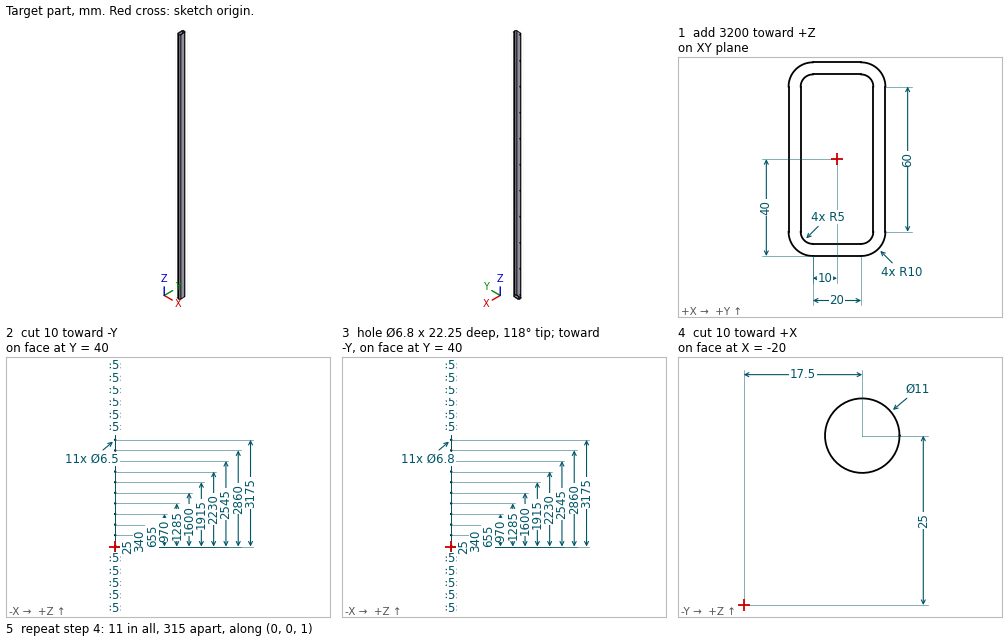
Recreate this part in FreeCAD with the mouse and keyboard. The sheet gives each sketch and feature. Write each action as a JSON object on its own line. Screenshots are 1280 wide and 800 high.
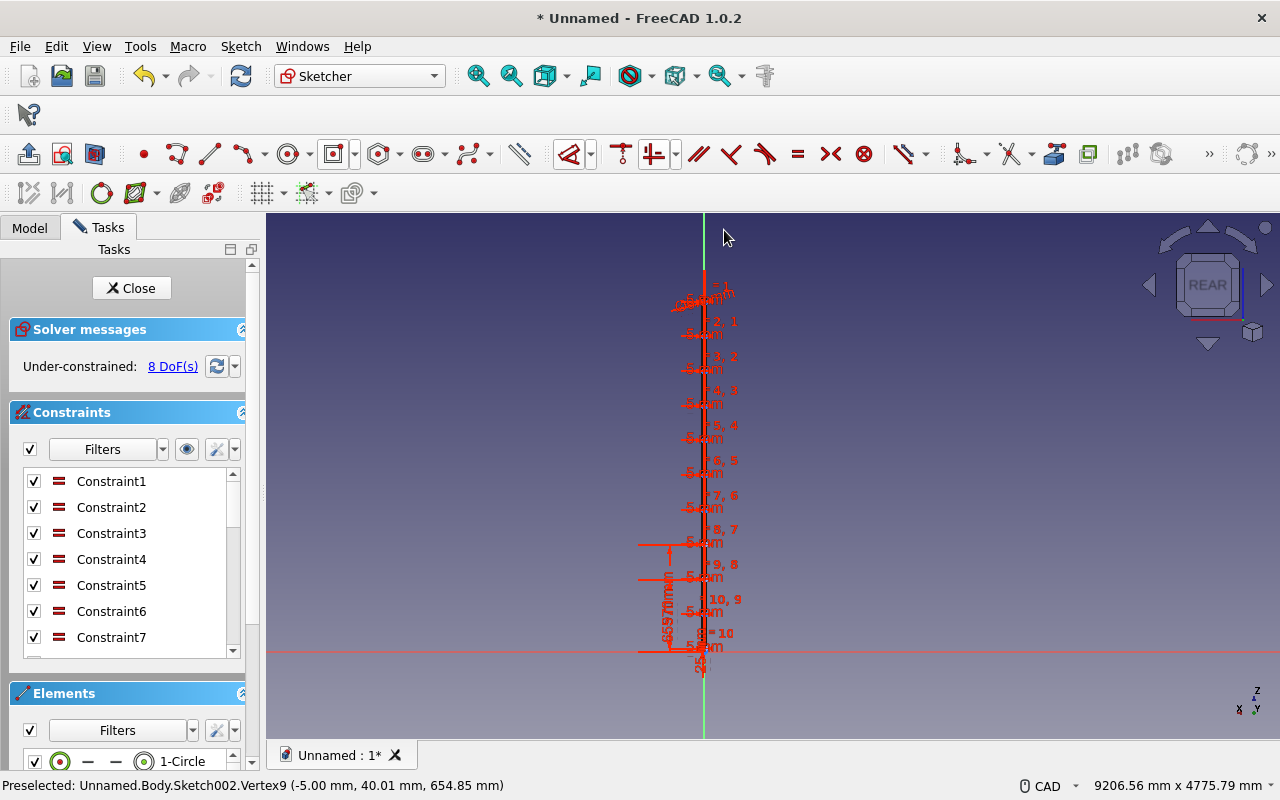
{"action": "left_click", "coordinate": [705, 614]}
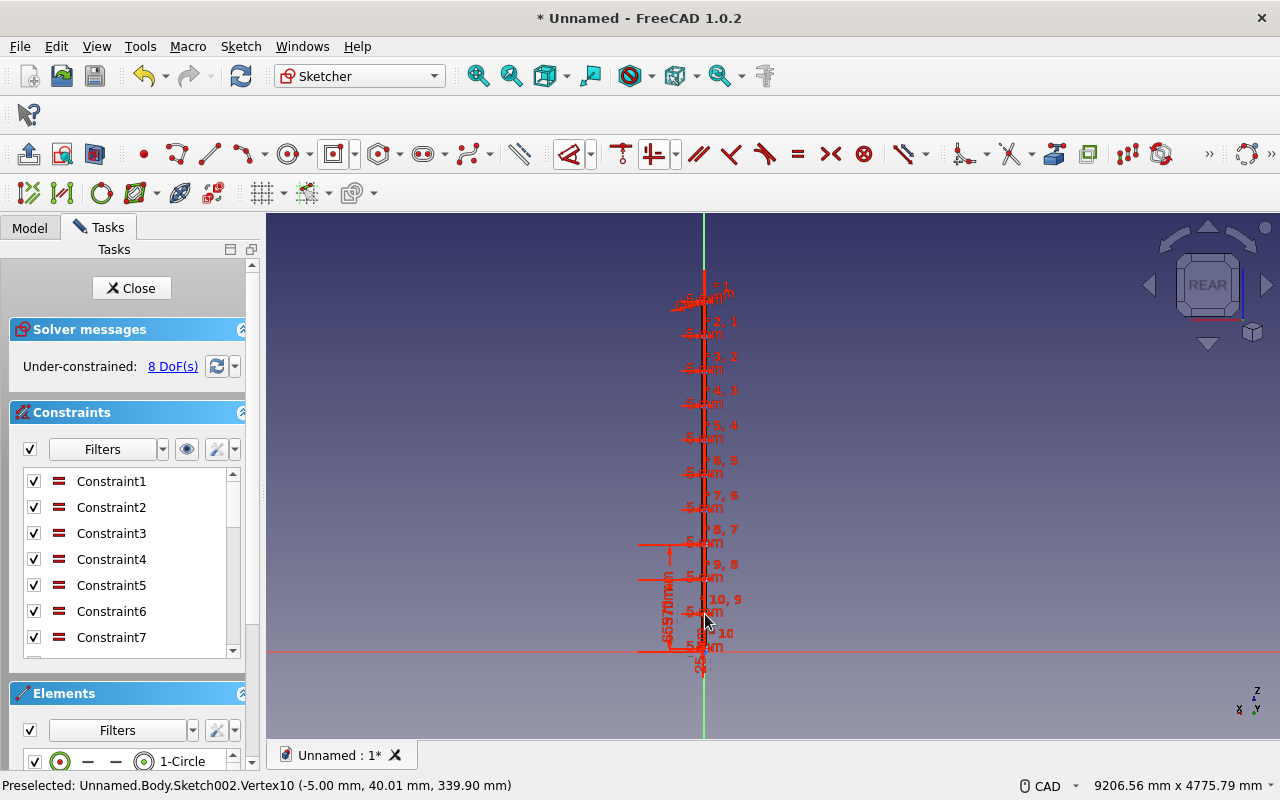
{"action": "left_click", "coordinate": [590, 154]}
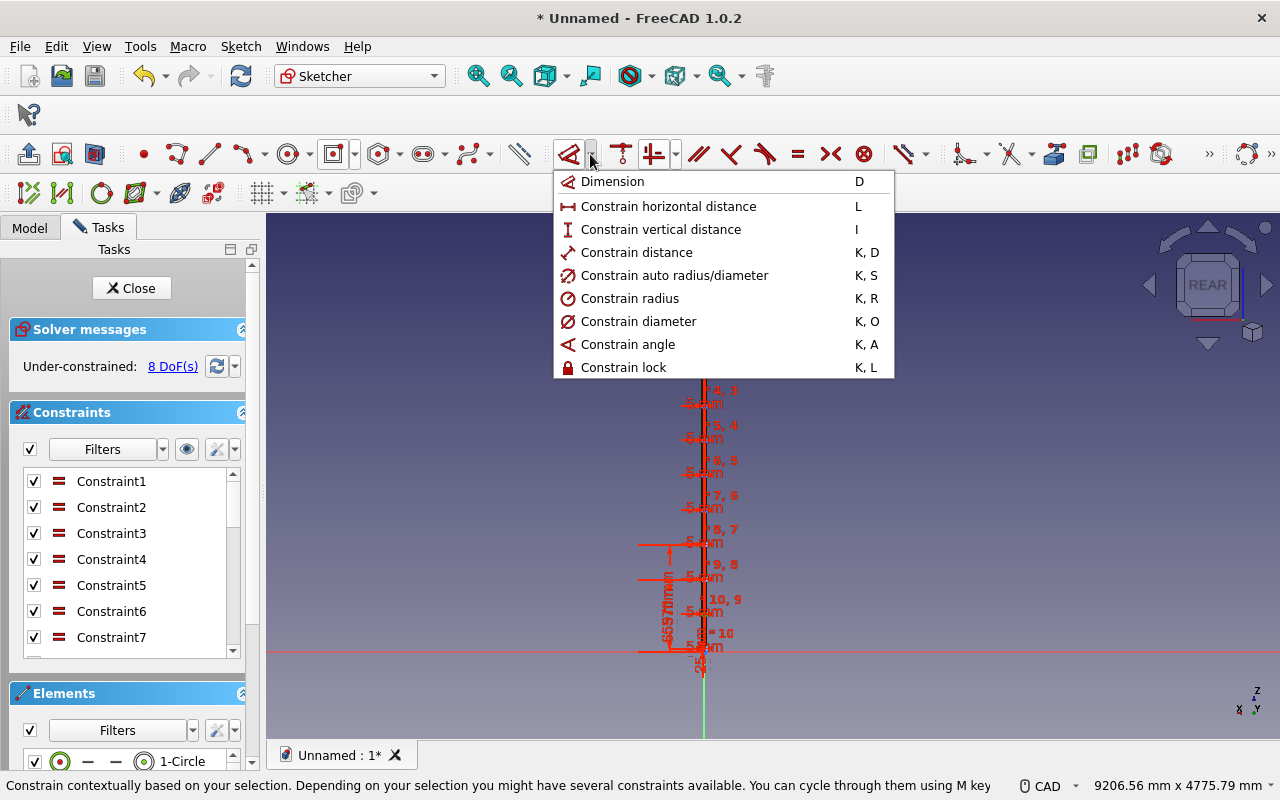
{"action": "left_click", "coordinate": [724, 230]}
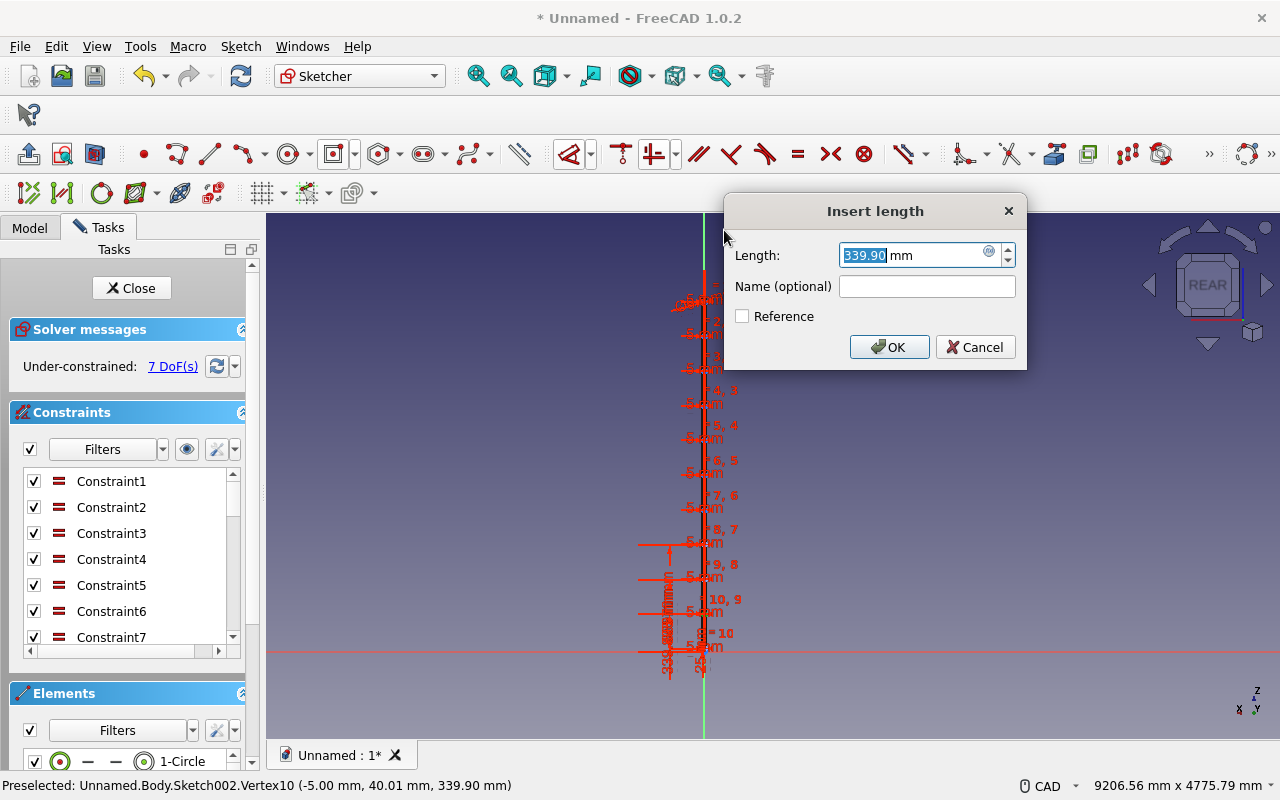
{"action": "type", "text": "340"}
{"action": "key", "text": "Return"}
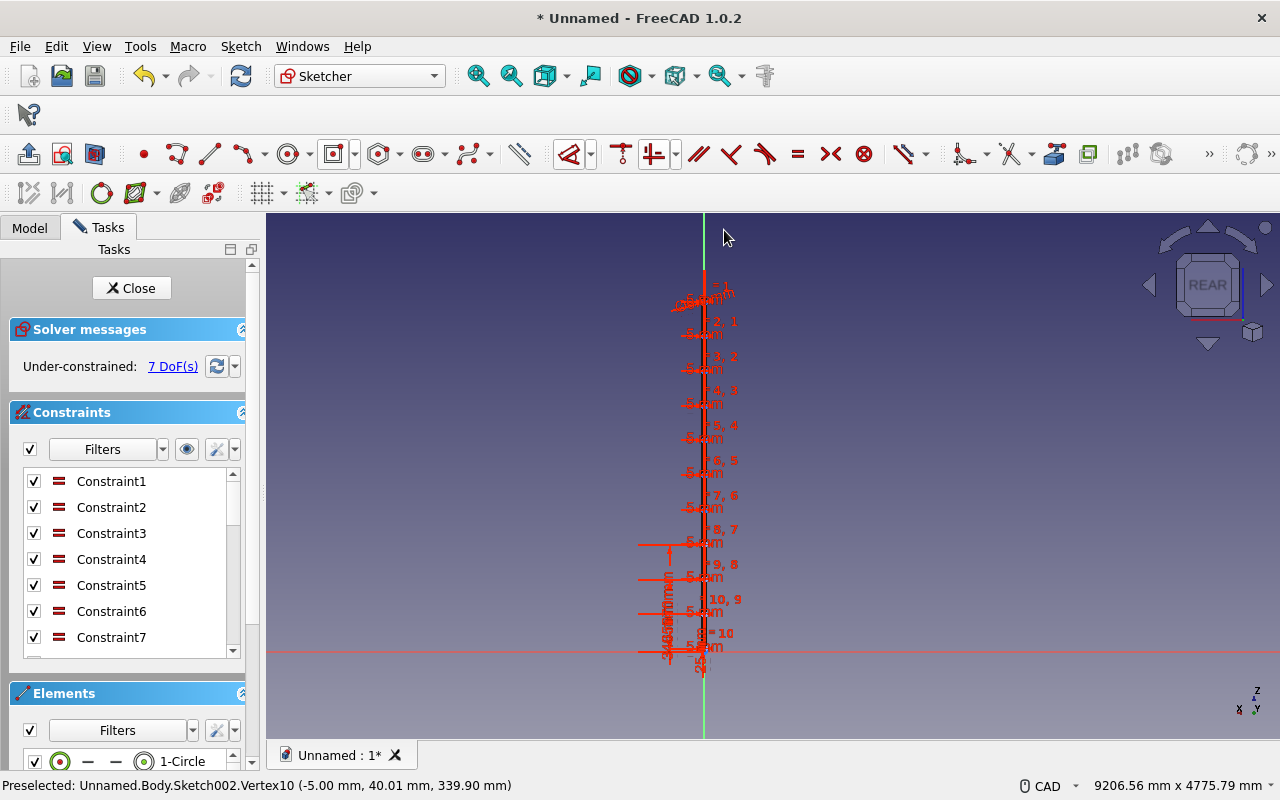
{"action": "left_click", "coordinate": [705, 302]}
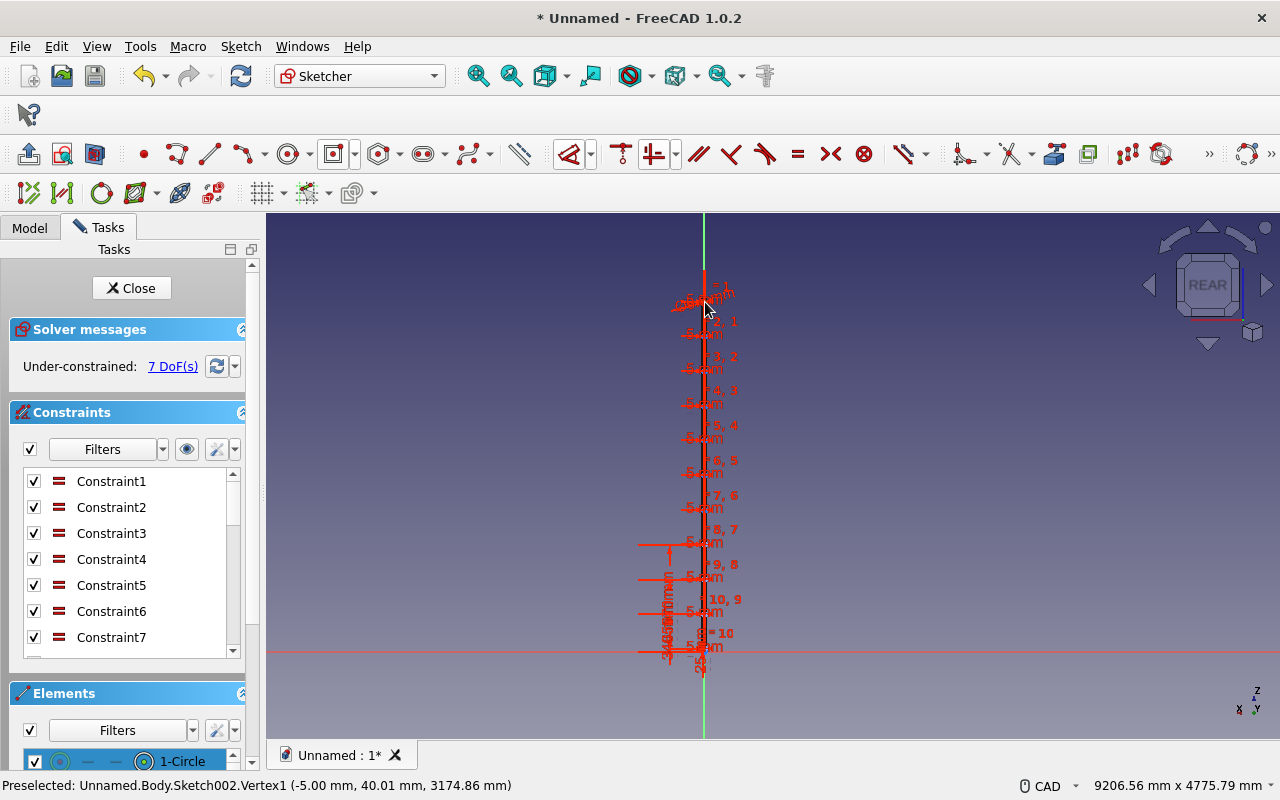
{"action": "key", "text": "i"}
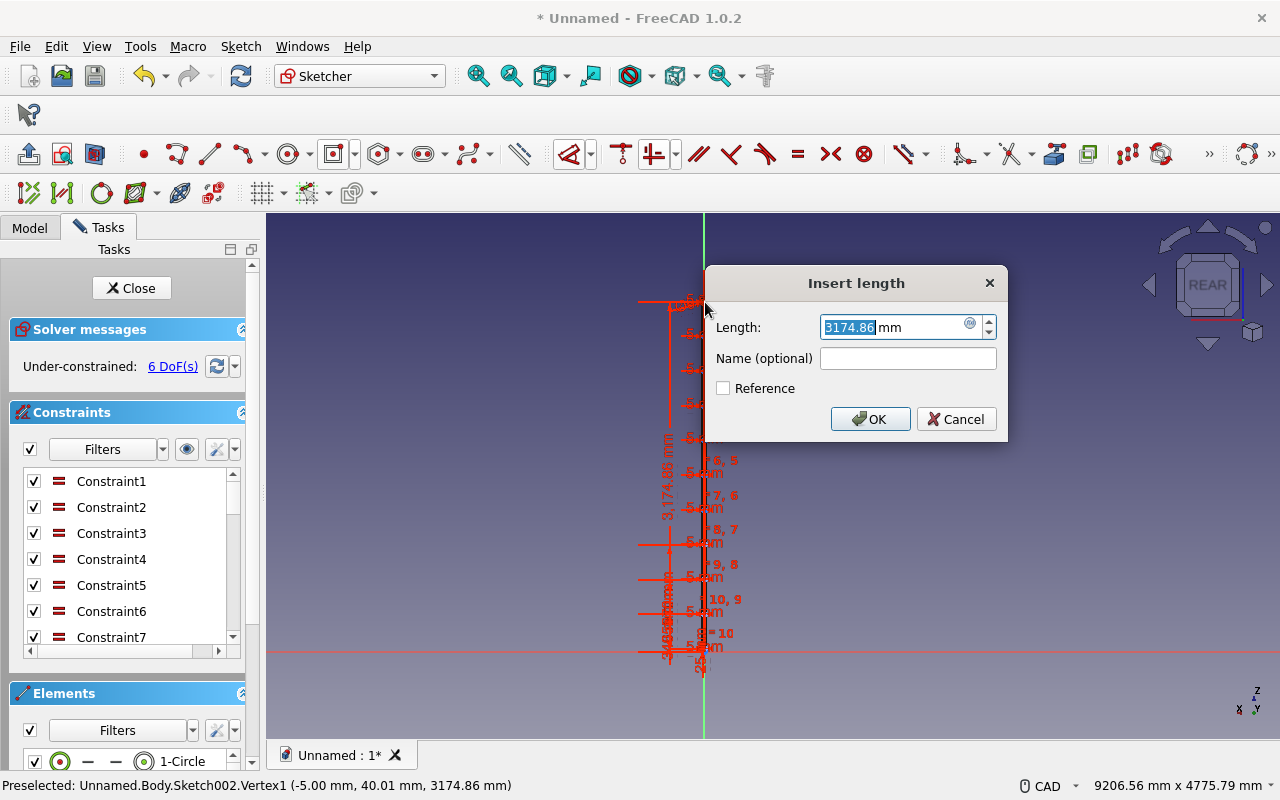
{"action": "type", "text": "3175"}
{"action": "key", "text": "Return"}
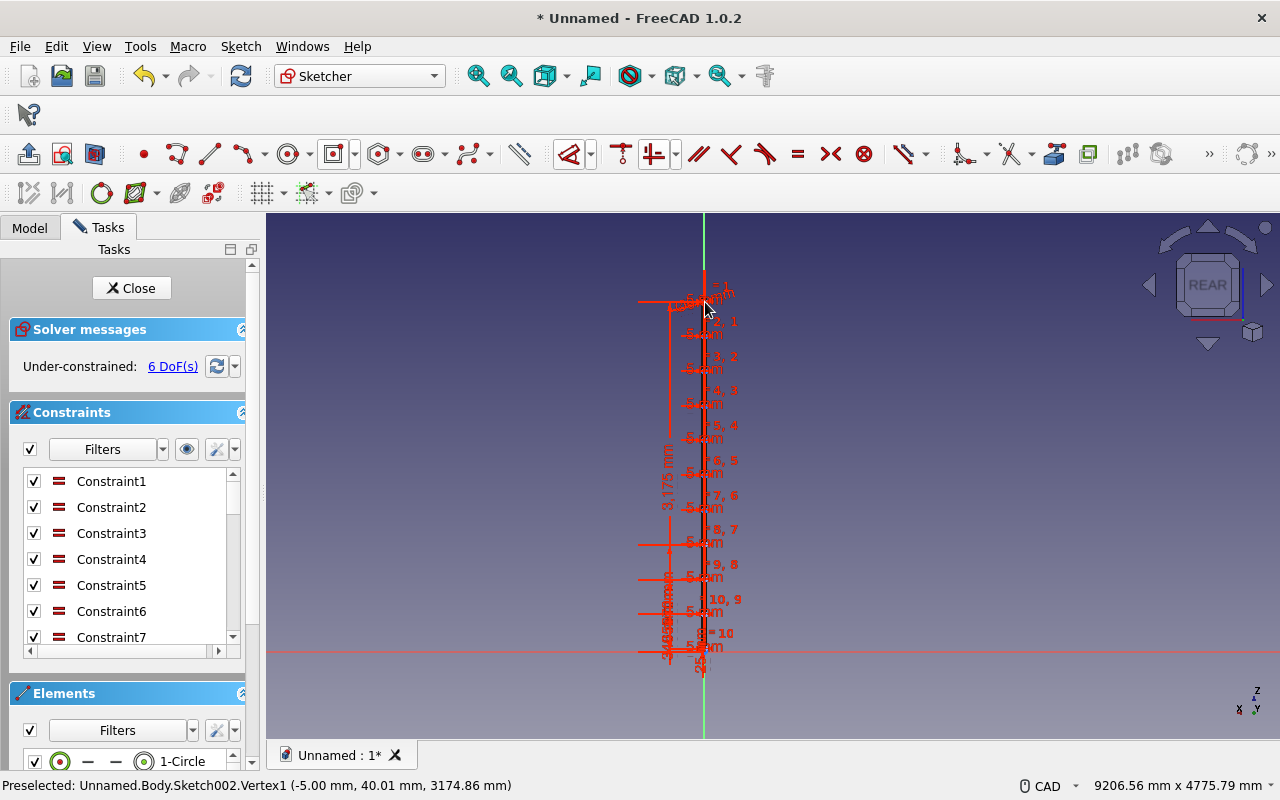
{"action": "left_click", "coordinate": [705, 337]}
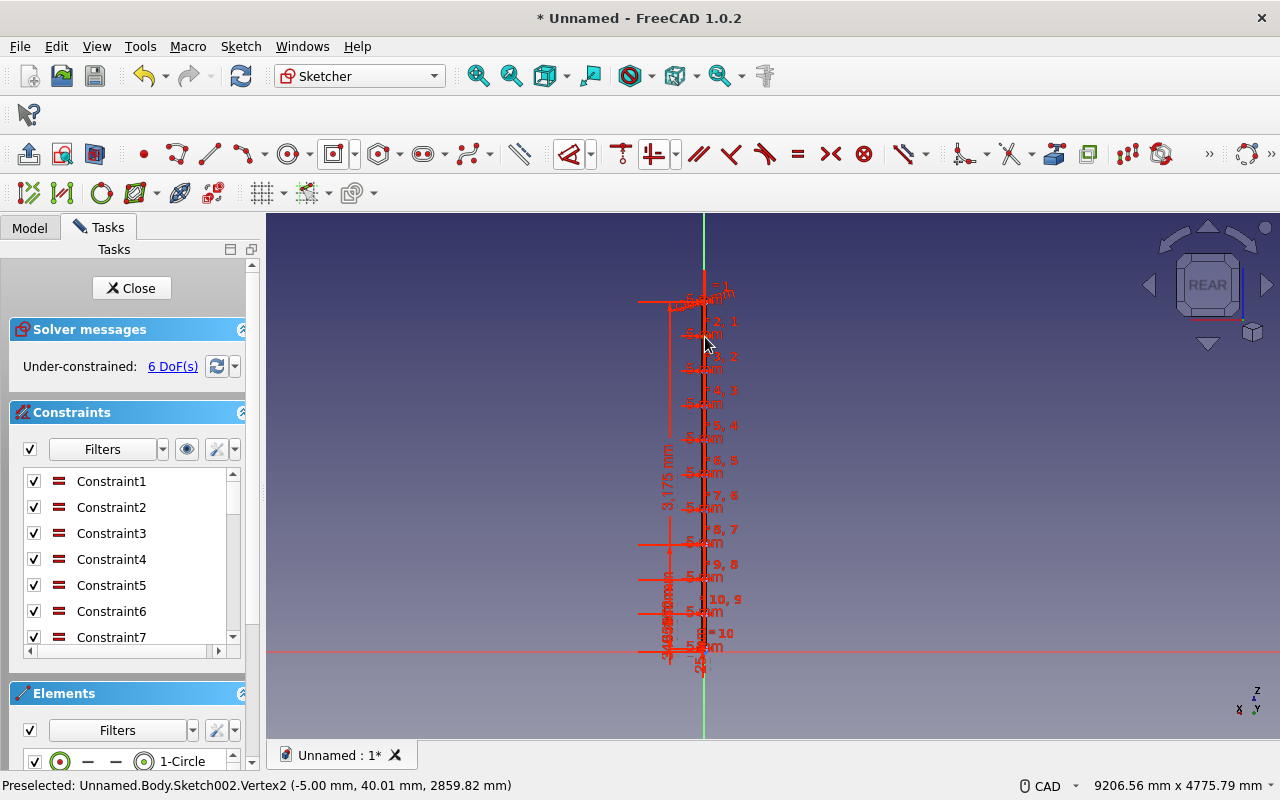
{"action": "left_click", "coordinate": [590, 154]}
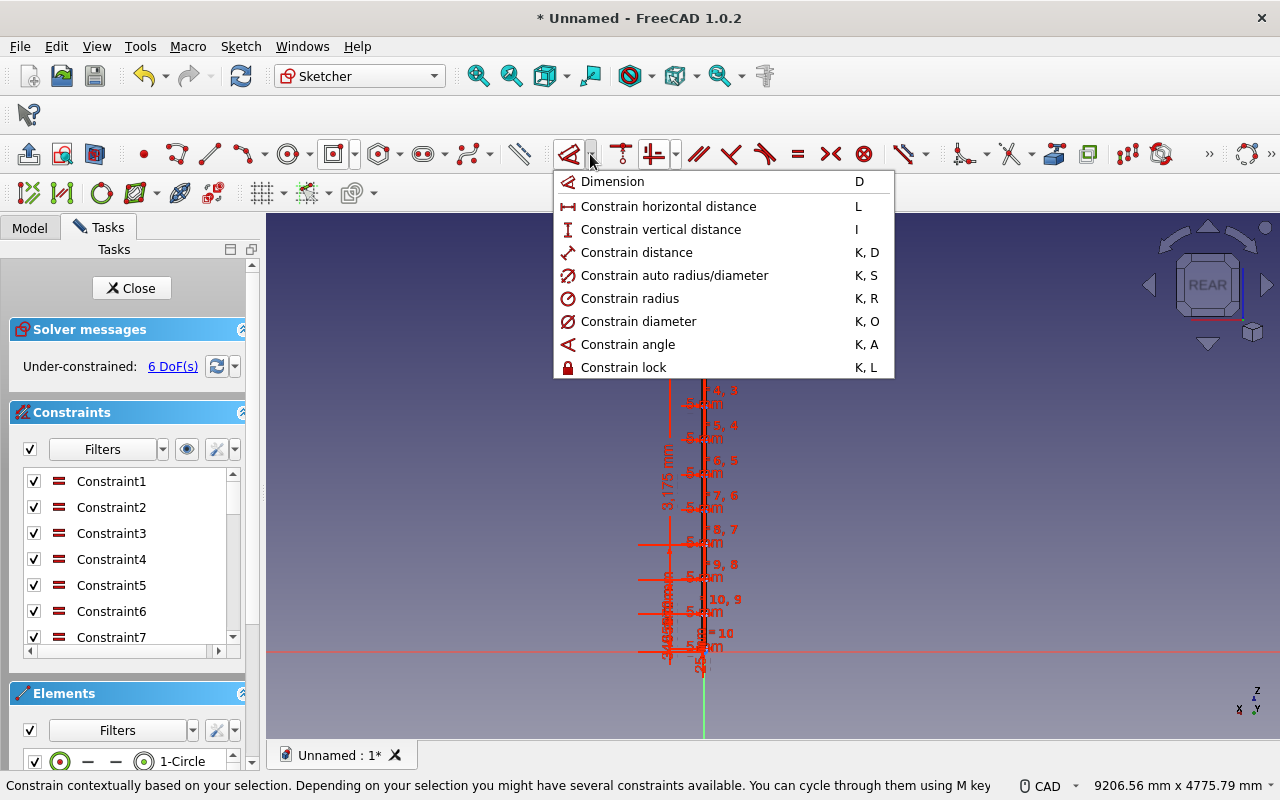
{"action": "left_click", "coordinate": [724, 230]}